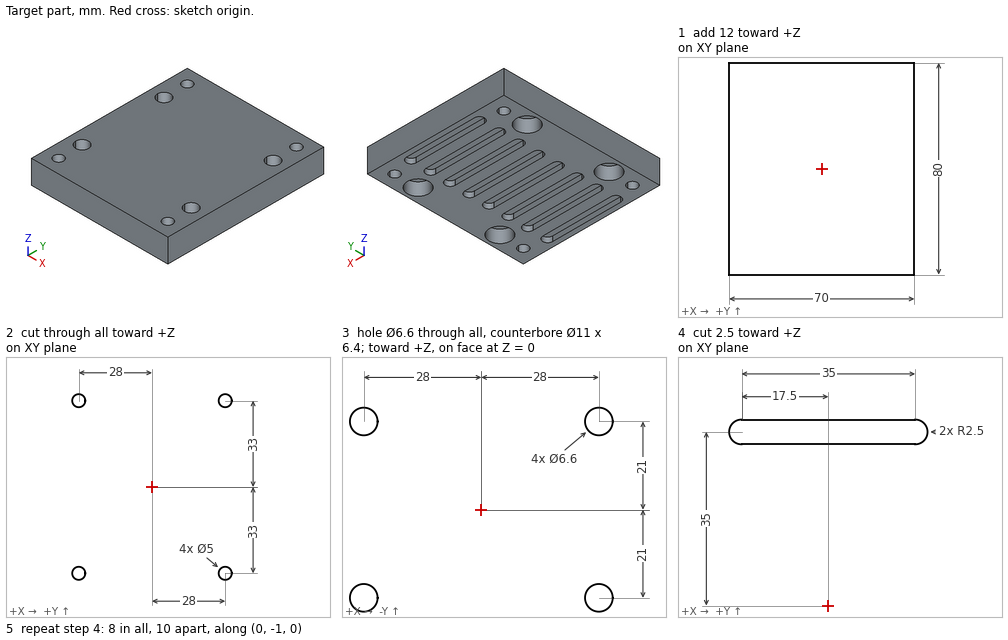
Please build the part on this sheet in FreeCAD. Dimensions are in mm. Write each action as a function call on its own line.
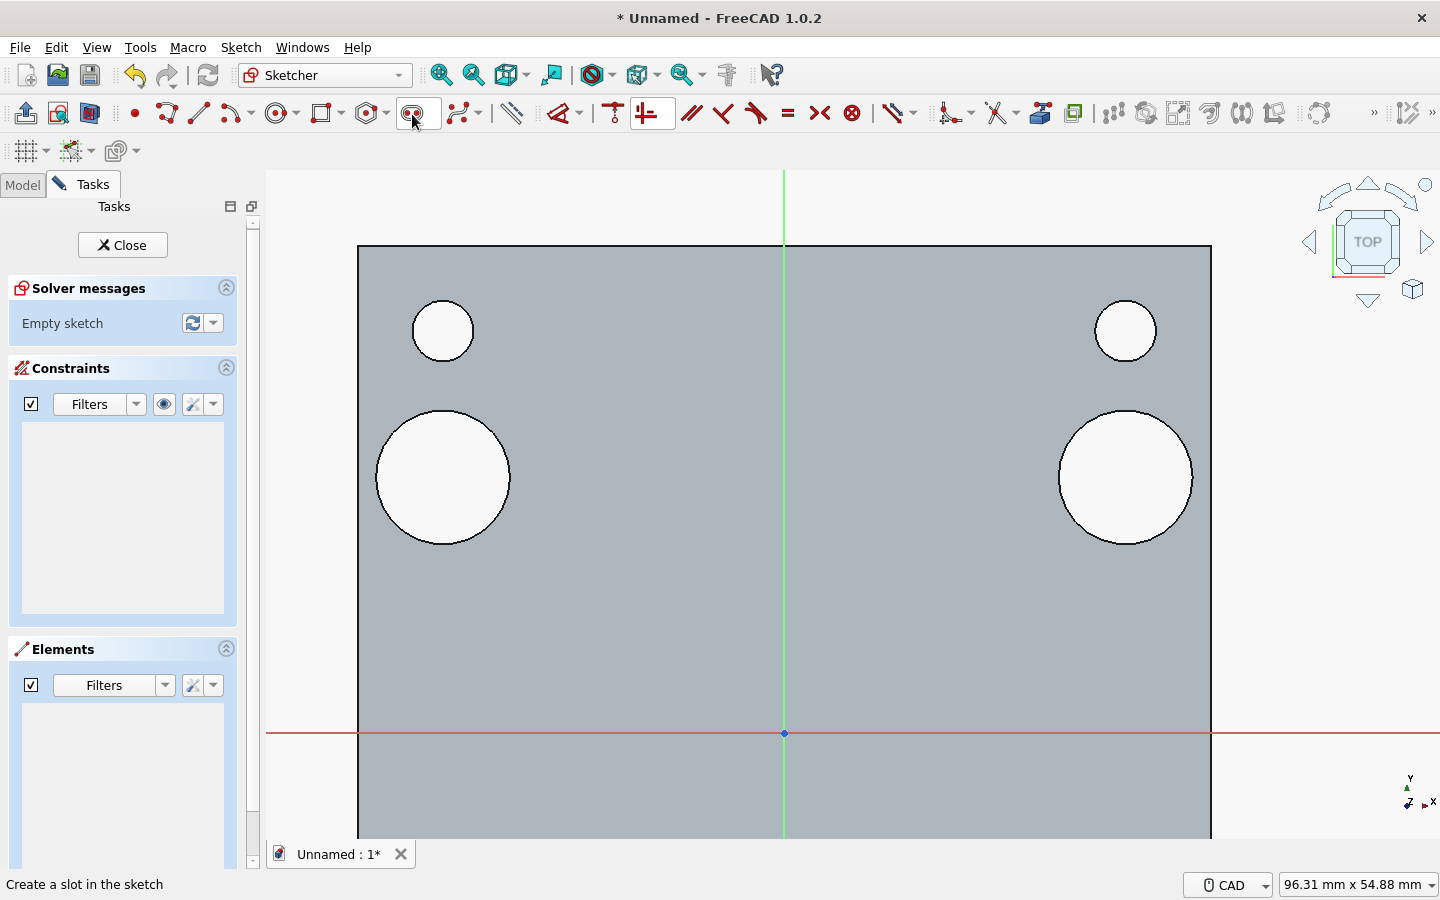
click(571, 307)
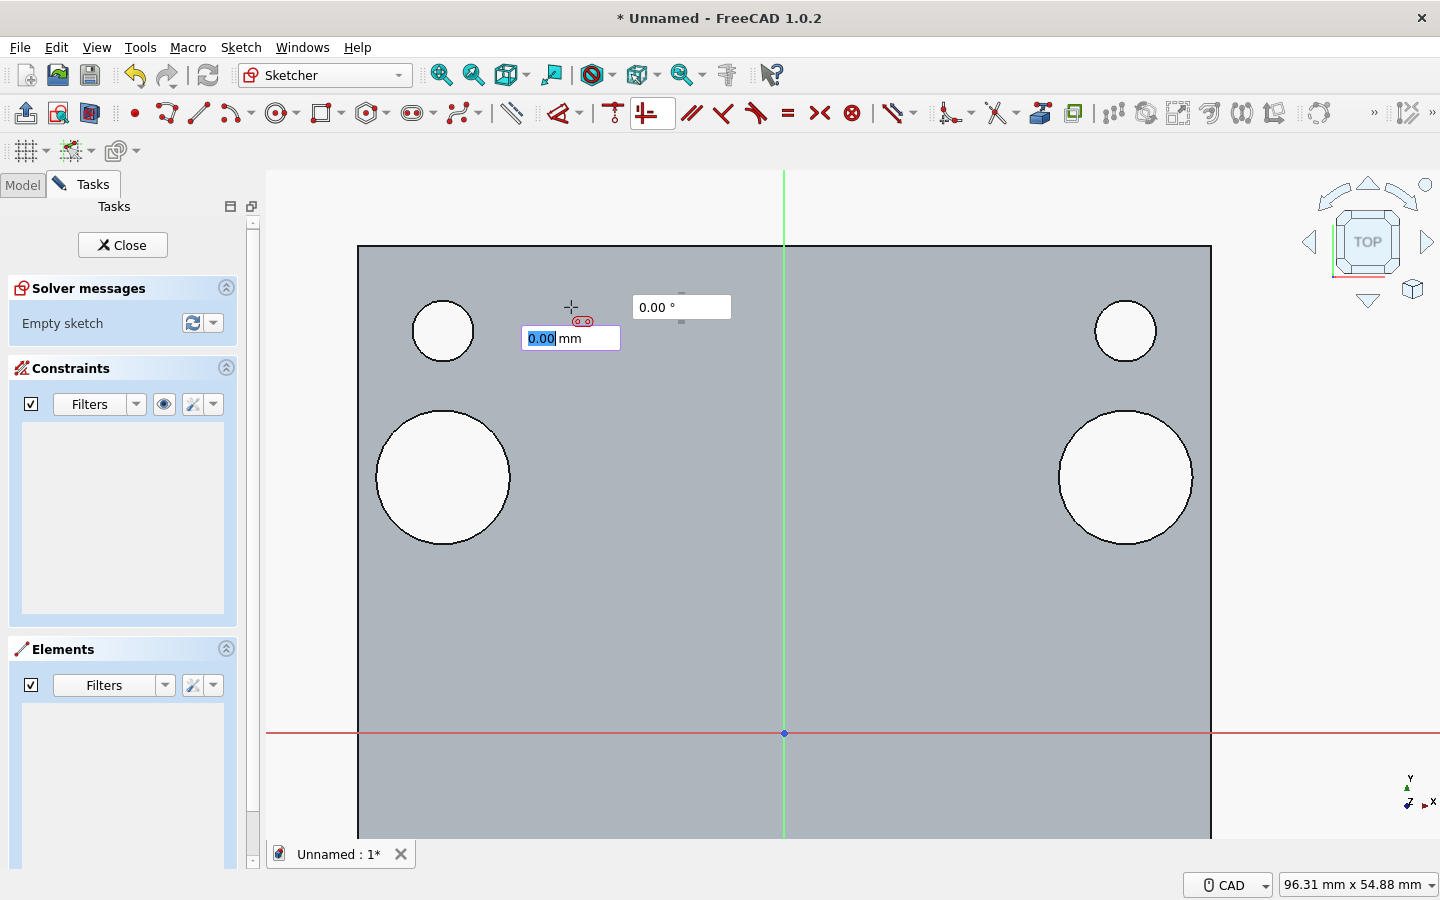
click(998, 307)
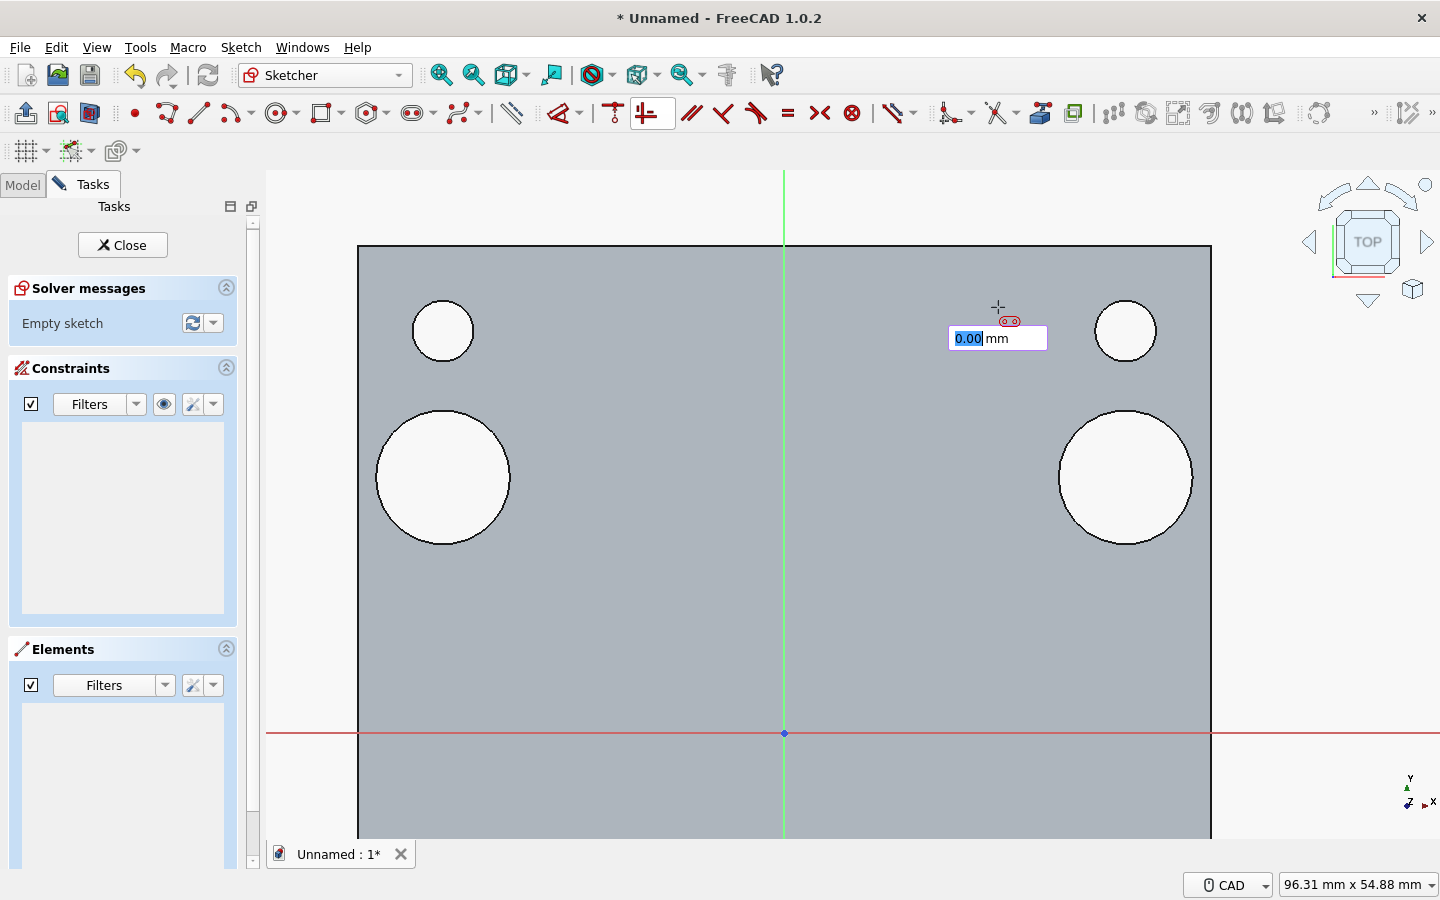
click(848, 337)
key(Escape)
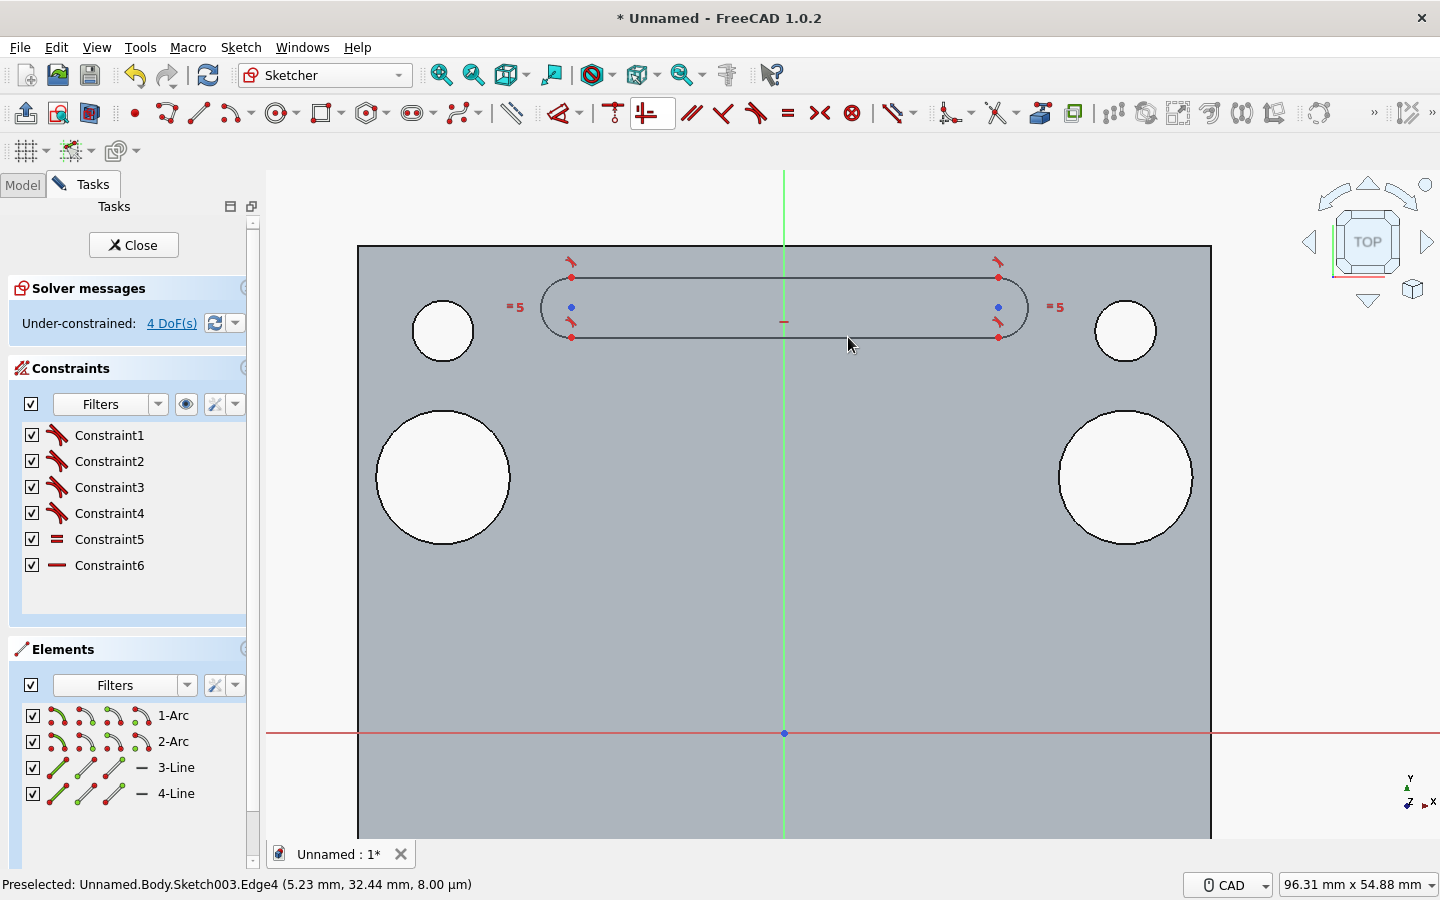
click(558, 114)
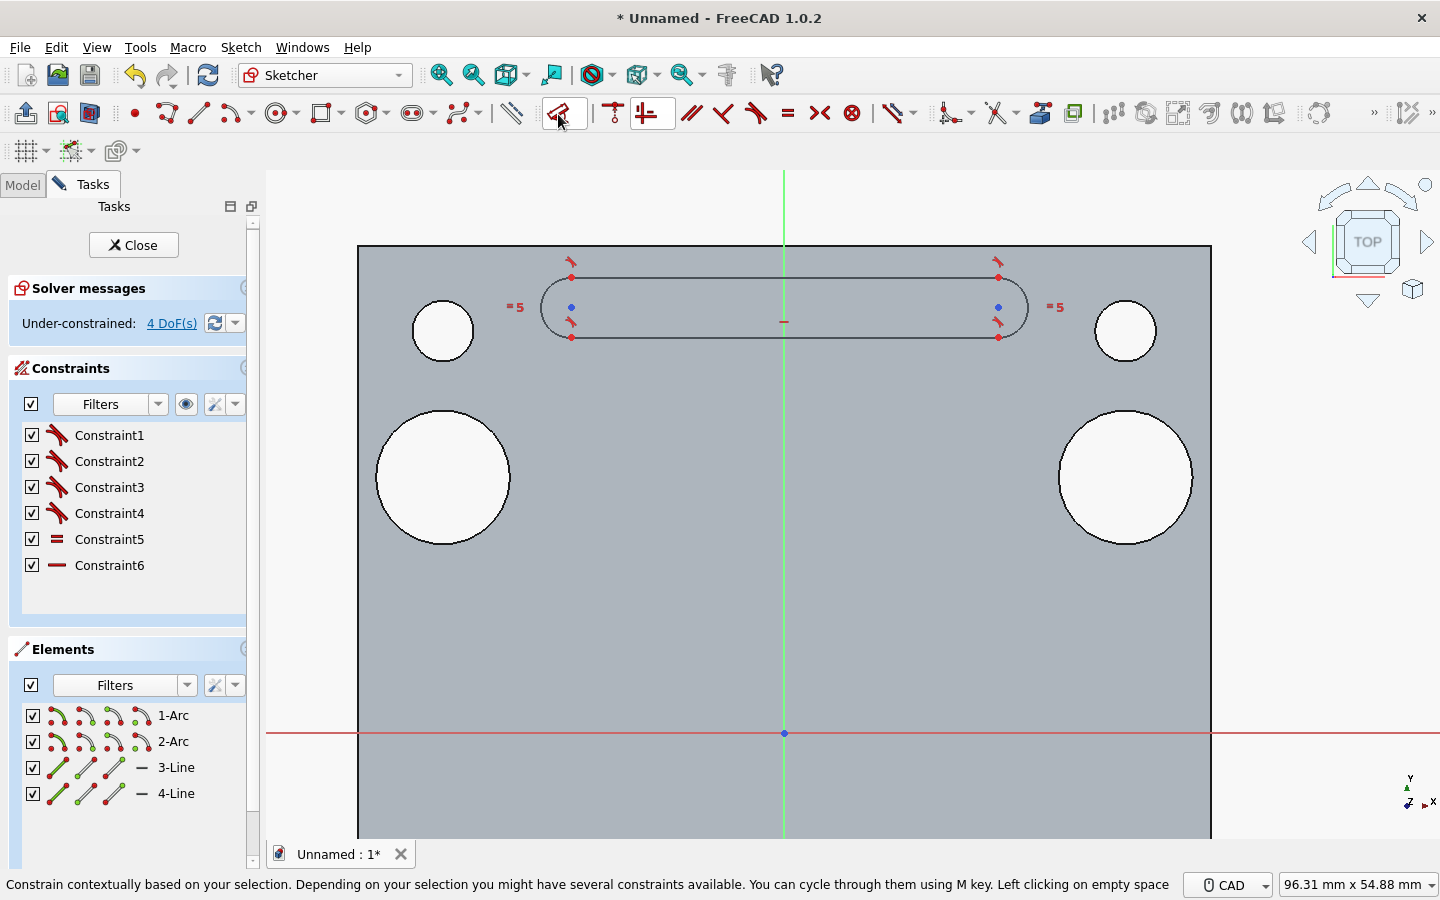
scroll(547, 290, up, 2)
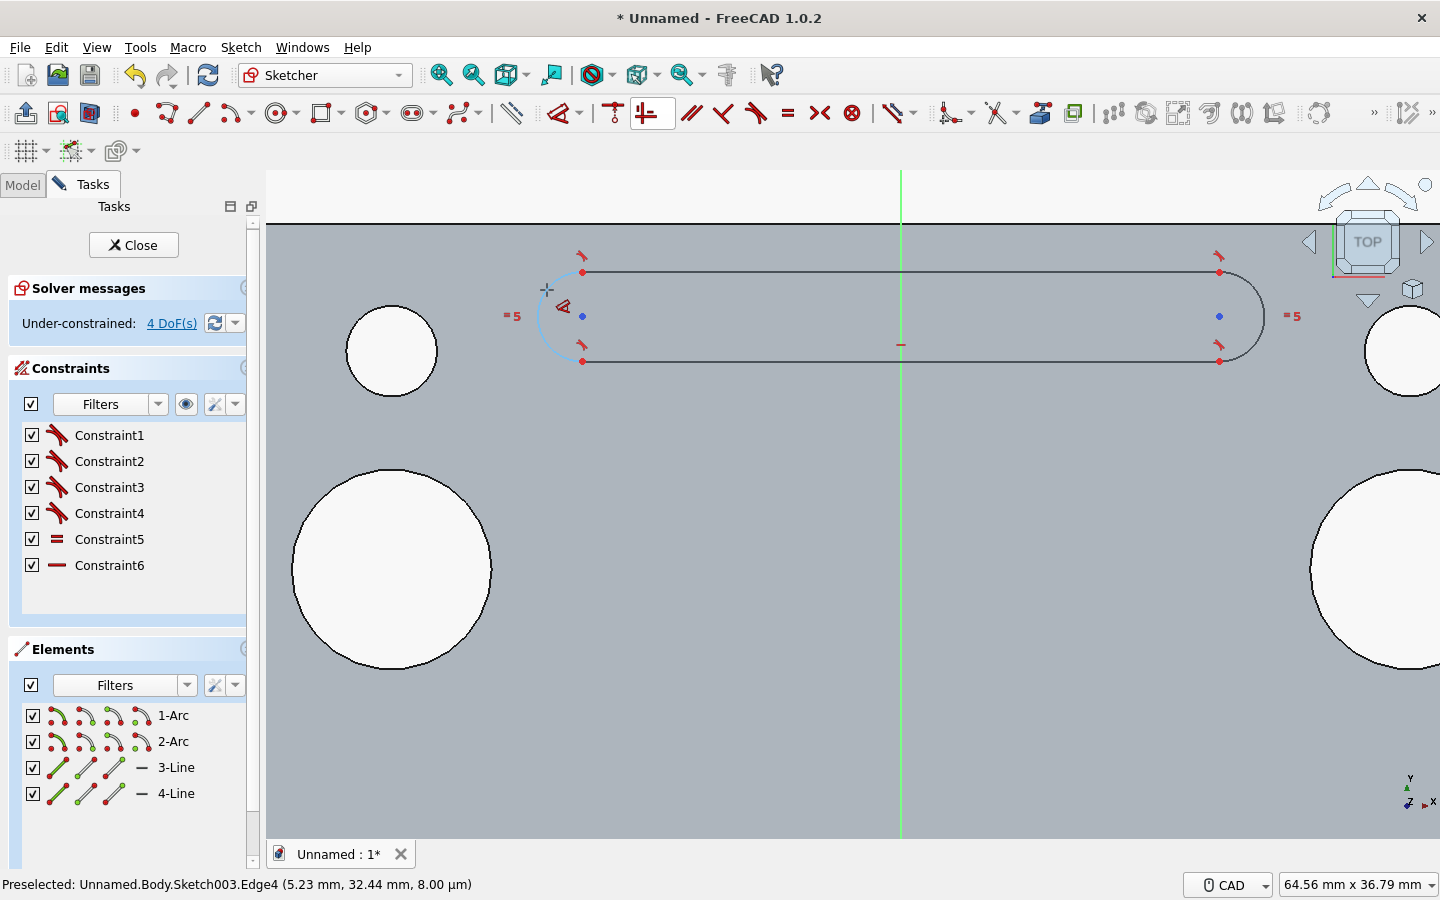
click(546, 290)
click(520, 271)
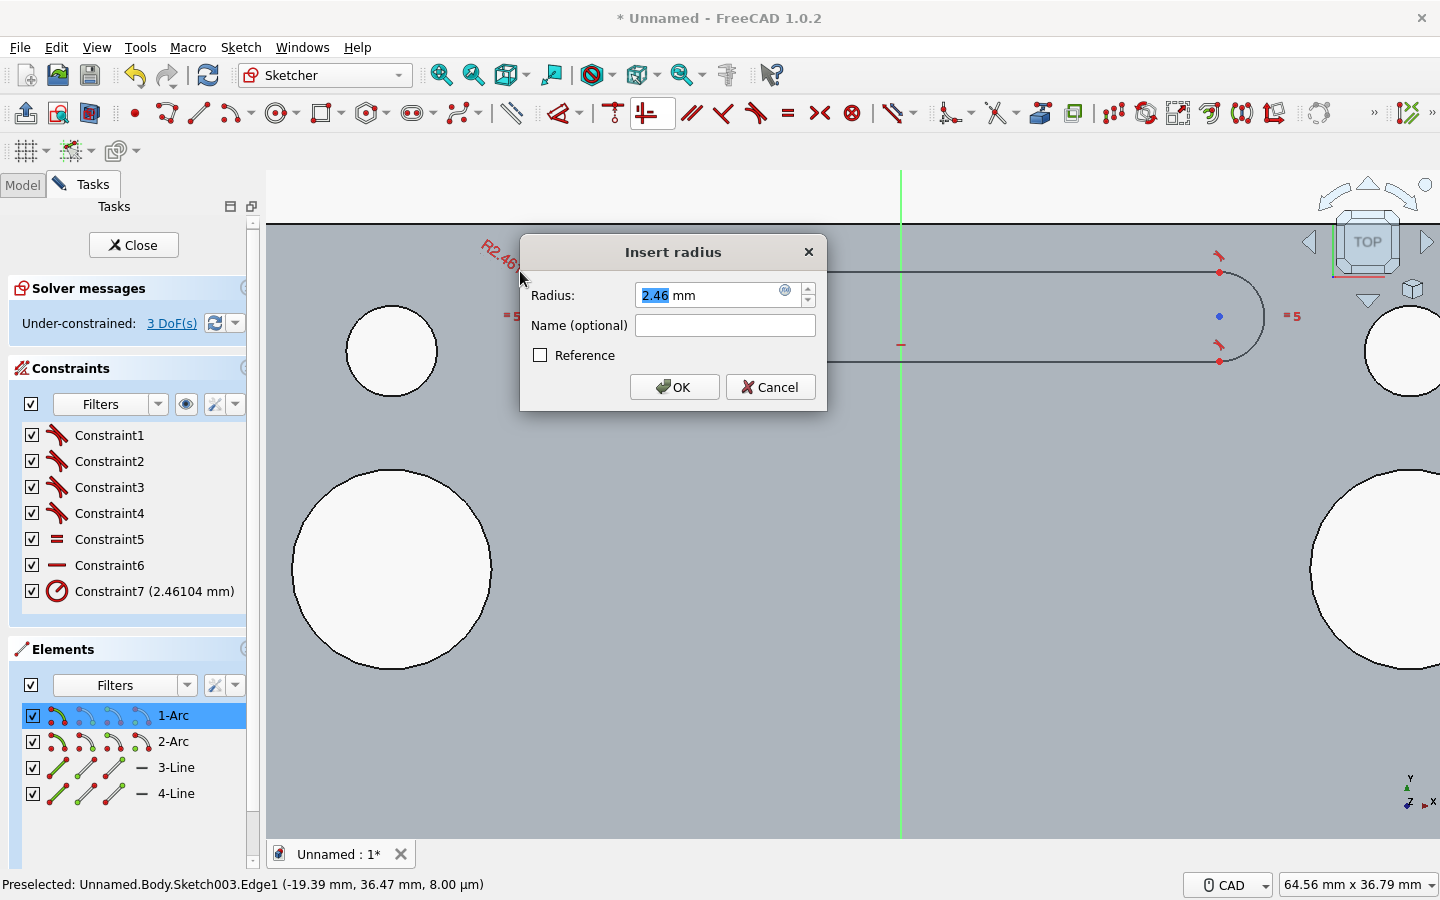
text(2.5)
key(Return)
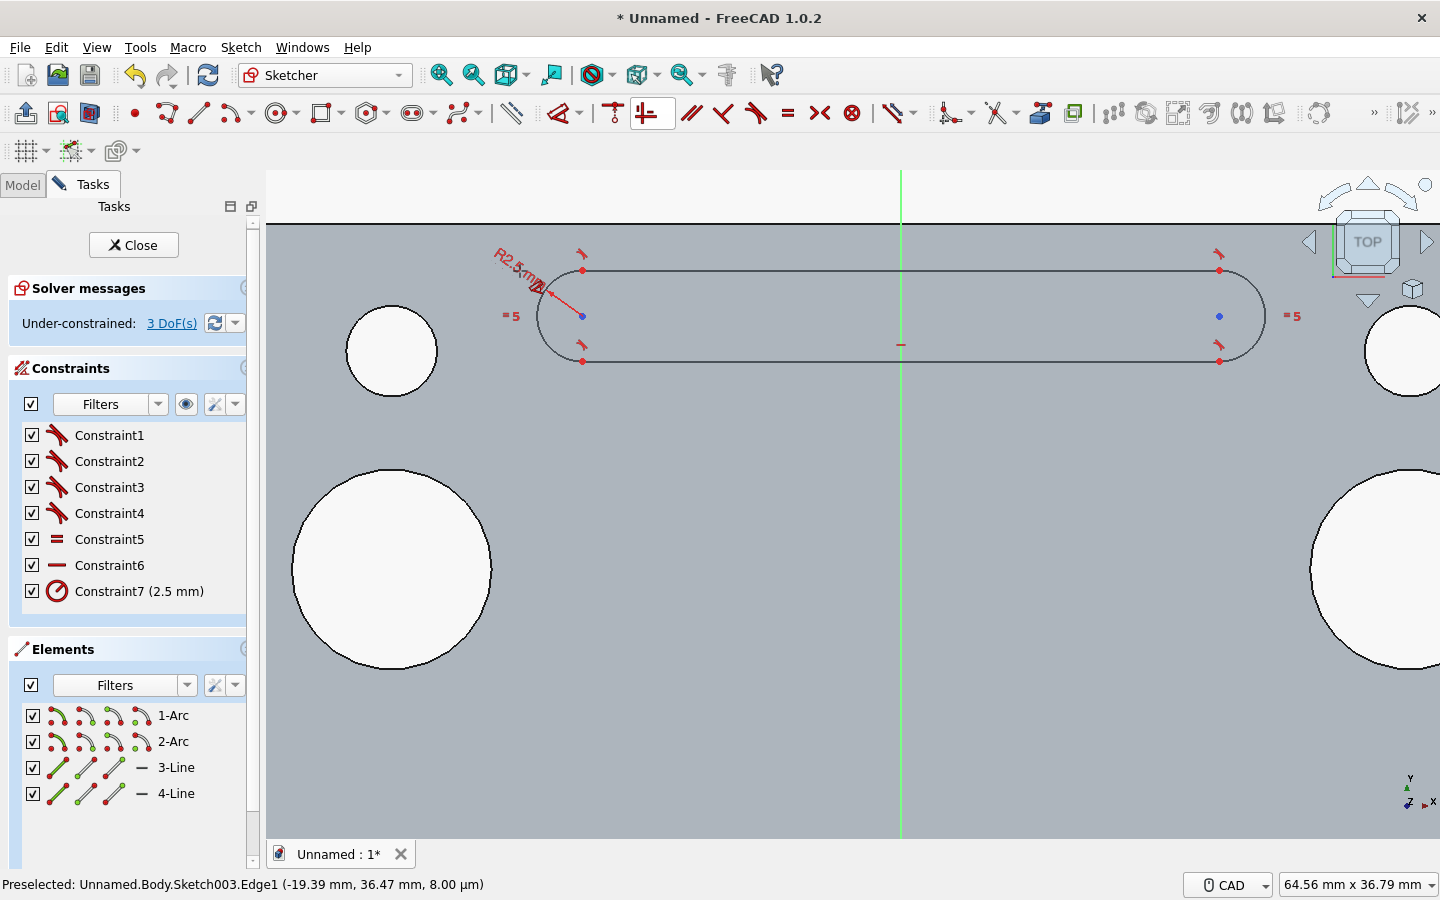
click(774, 271)
click(755, 237)